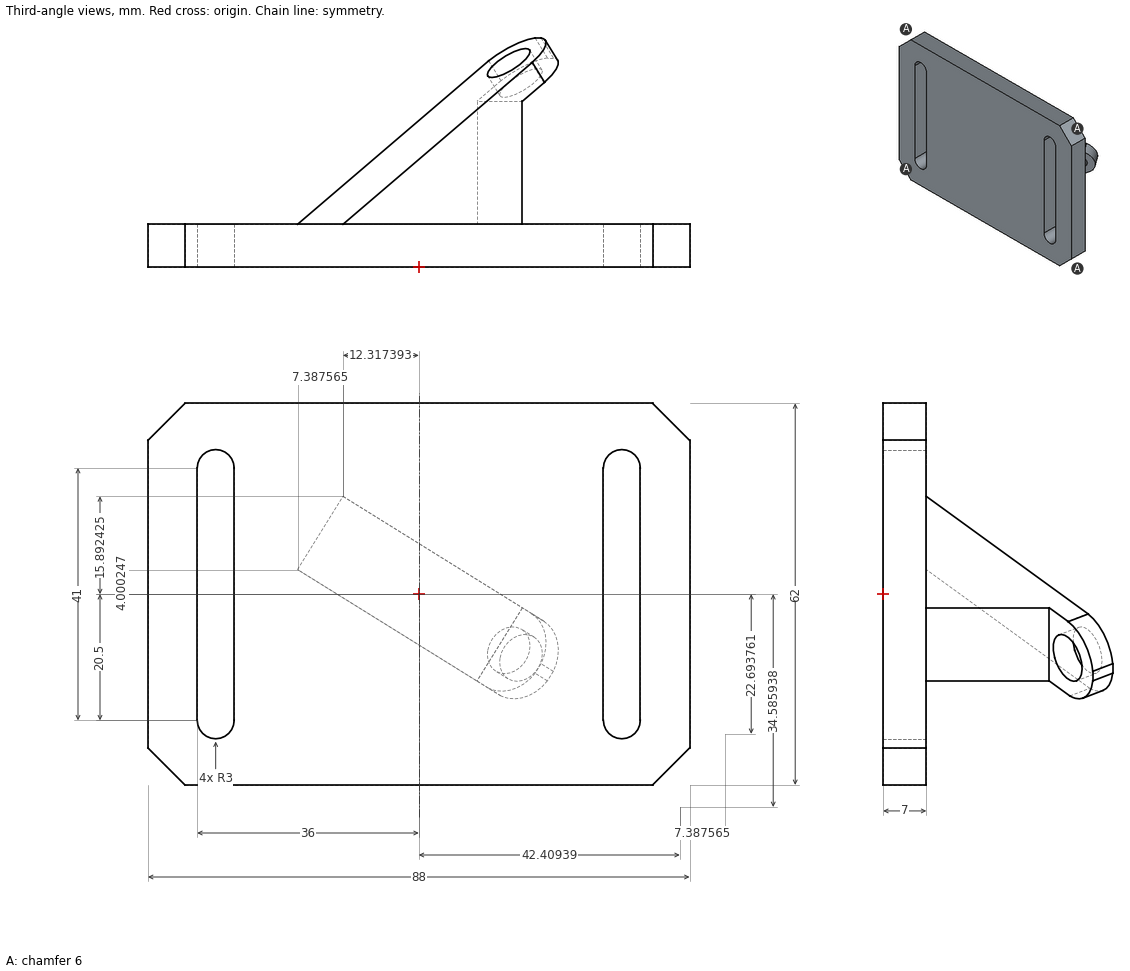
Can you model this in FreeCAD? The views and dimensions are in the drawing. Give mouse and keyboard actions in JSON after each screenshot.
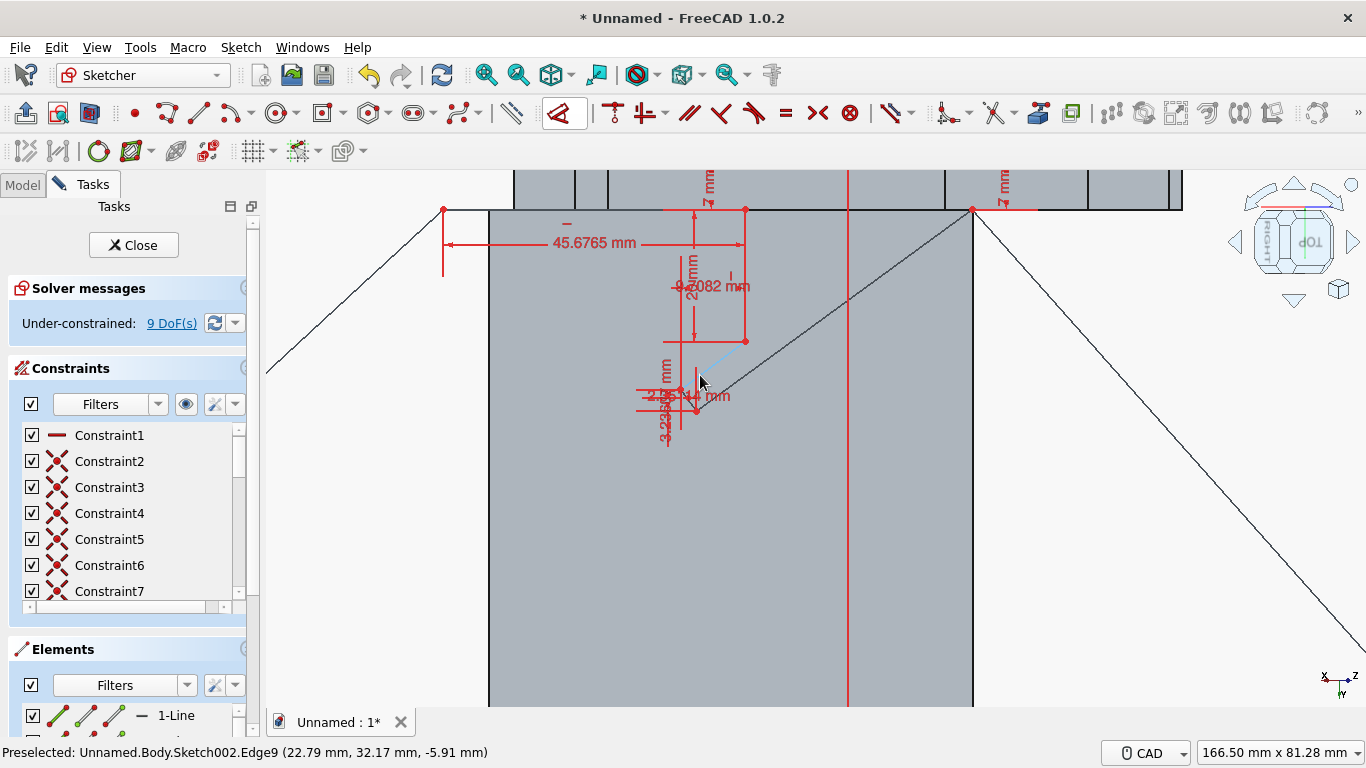
{"action": "left_click", "coordinate": [700, 375]}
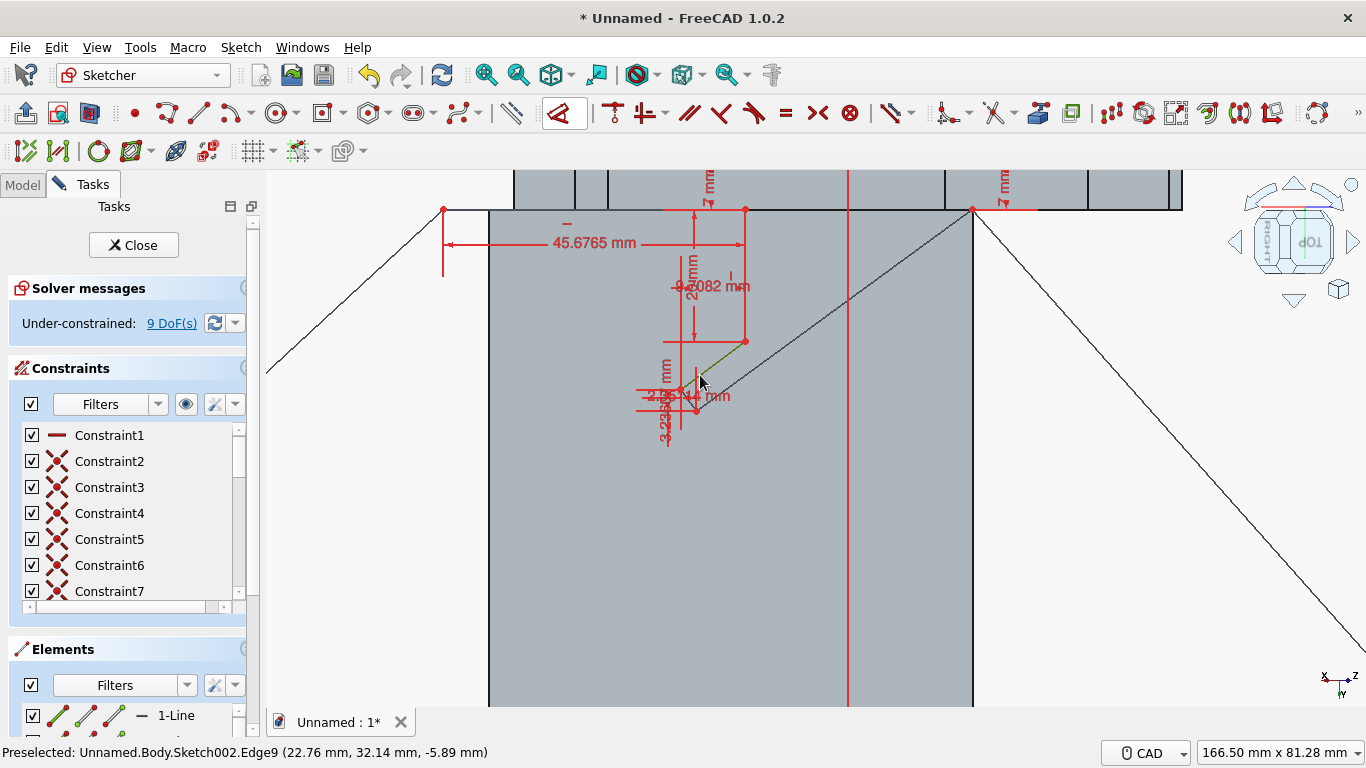
{"action": "left_click", "coordinate": [582, 114]}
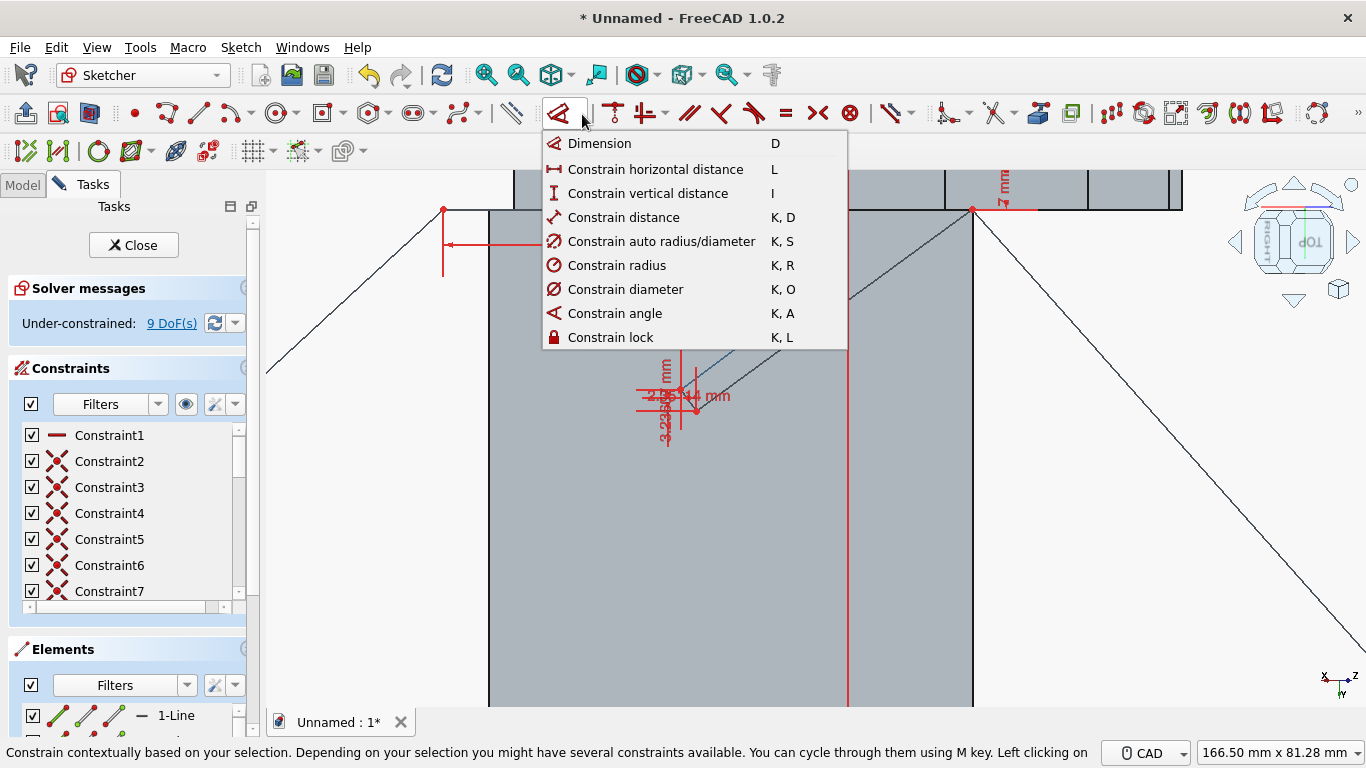
{"action": "left_click", "coordinate": [695, 193]}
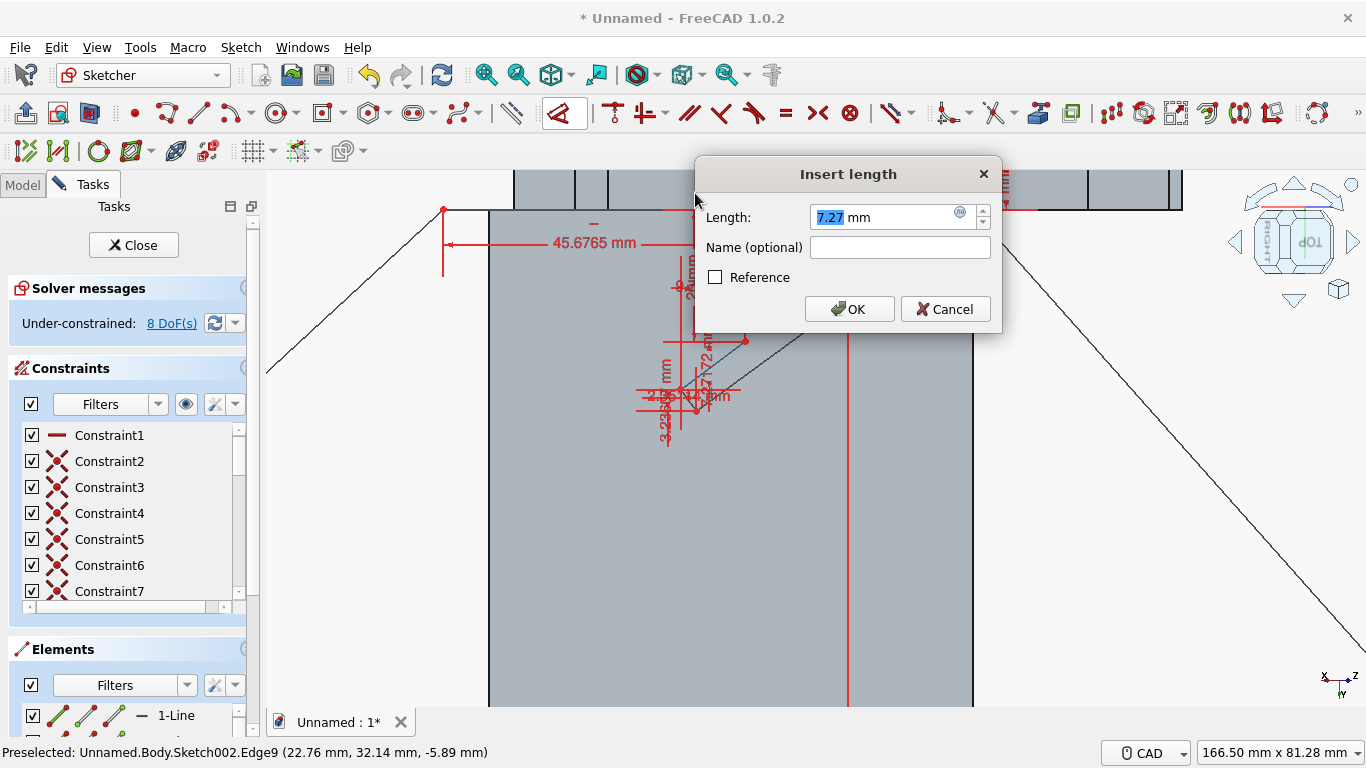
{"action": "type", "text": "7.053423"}
{"action": "key", "text": "Return"}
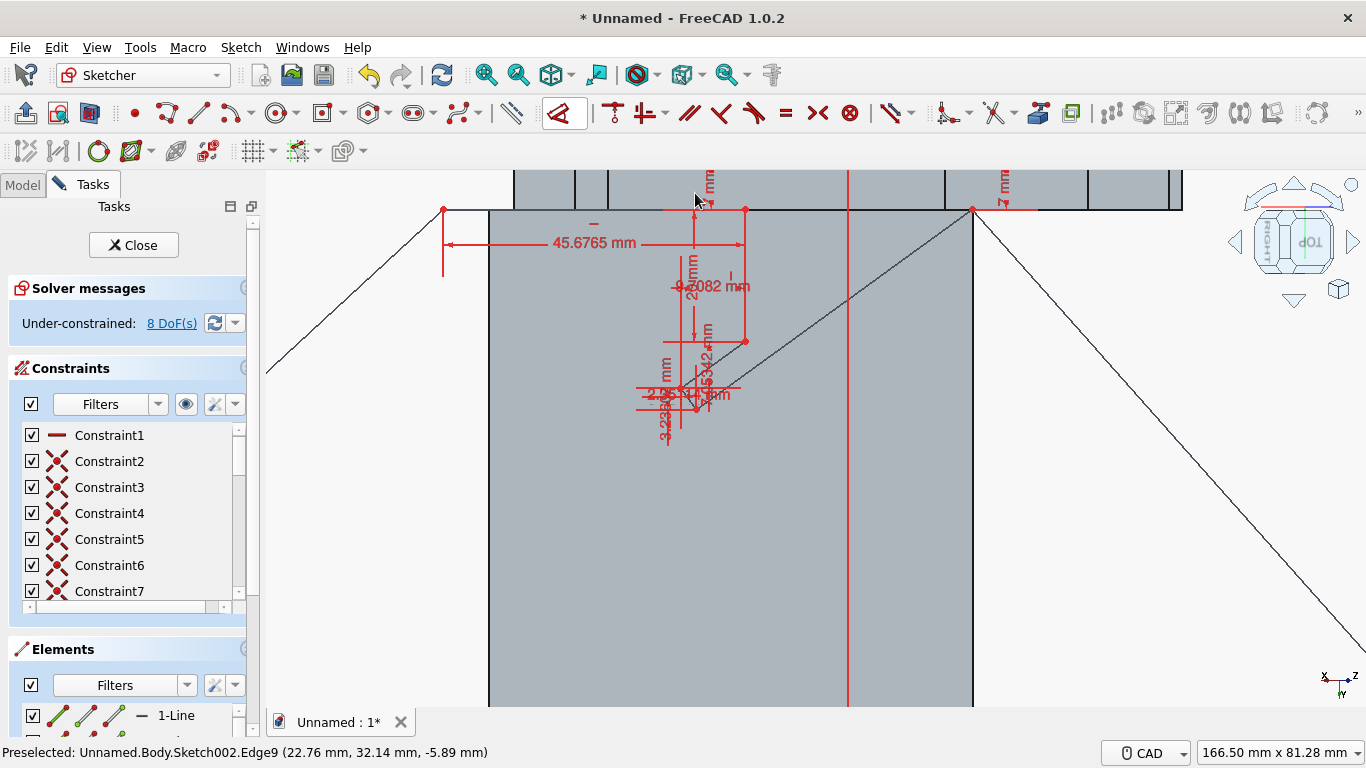
{"action": "left_click", "coordinate": [745, 210]}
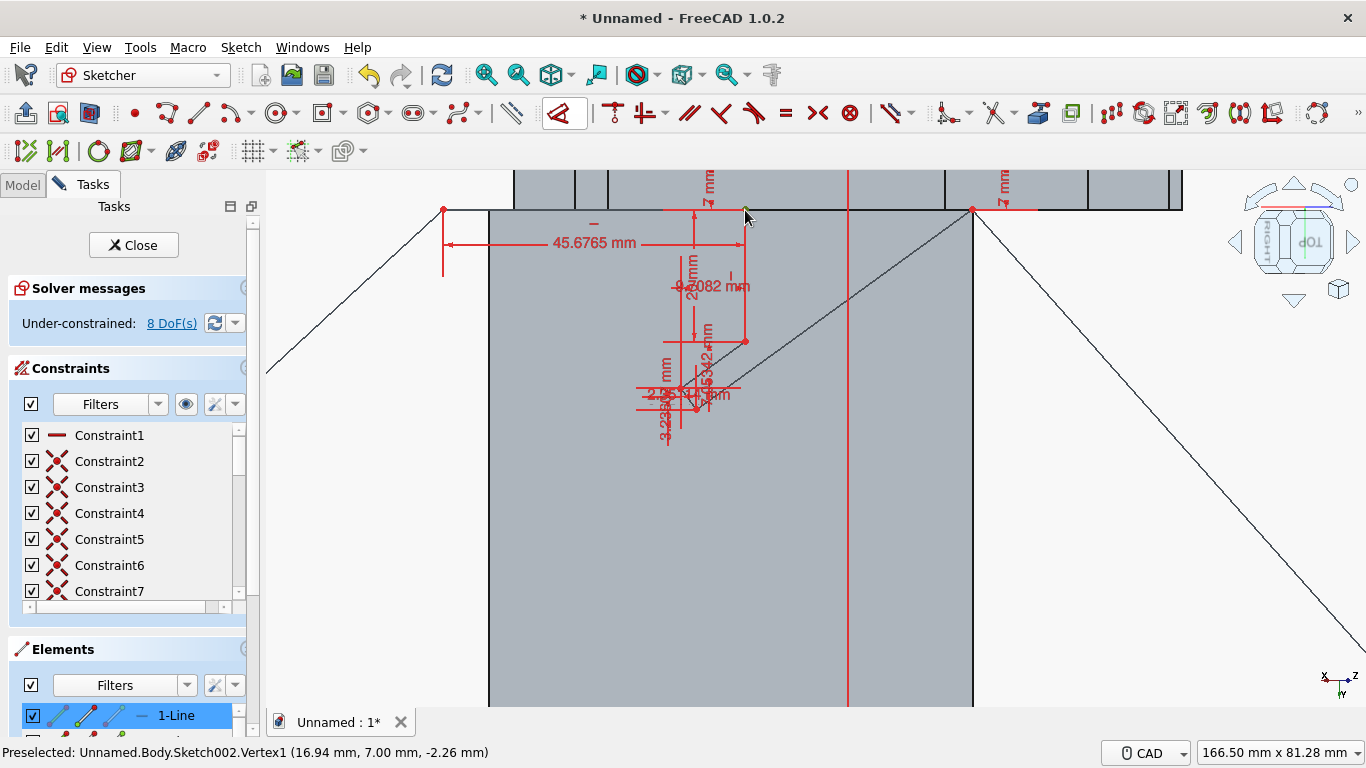
{"action": "left_click", "coordinate": [582, 114]}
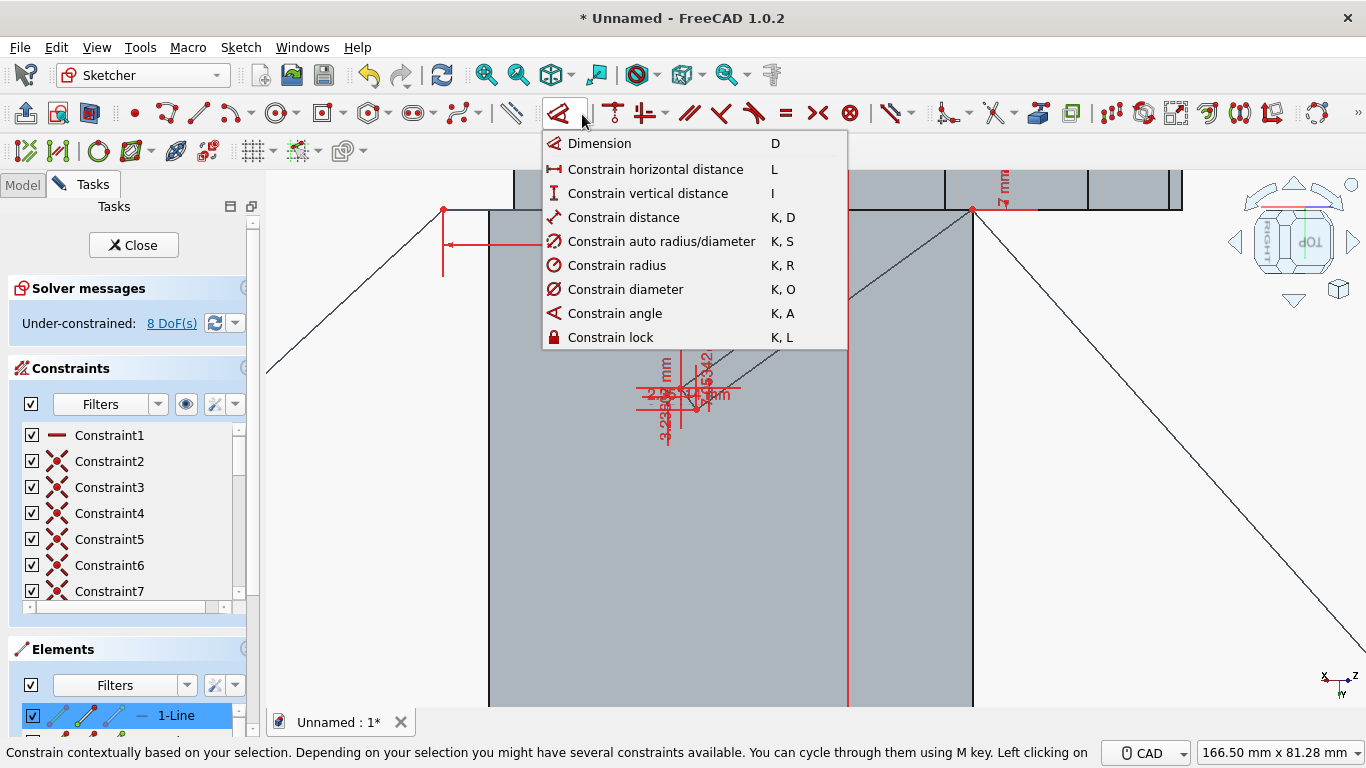
{"action": "left_click", "coordinate": [695, 169]}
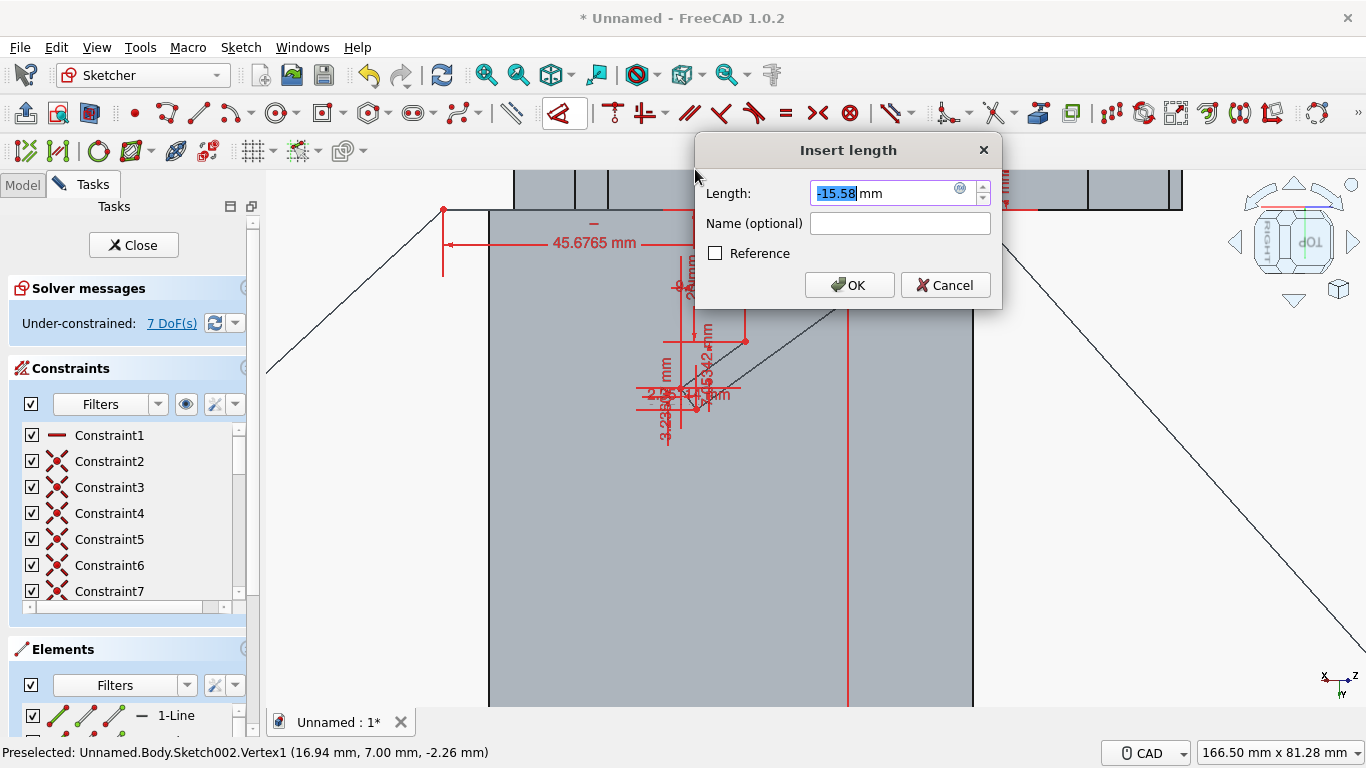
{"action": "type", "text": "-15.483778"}
{"action": "key", "text": "Return"}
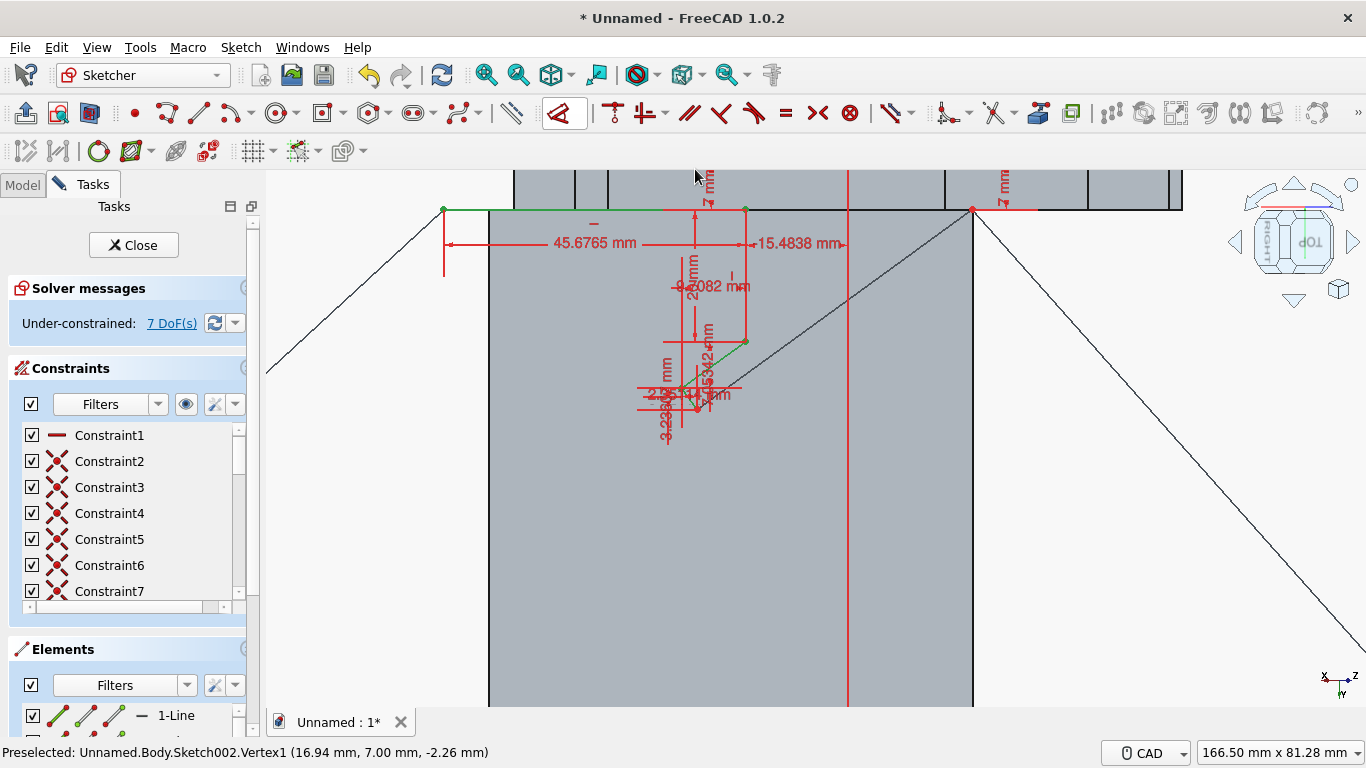
{"action": "scroll", "coordinate": [701, 375], "scroll_direction": "down", "scroll_amount": 4}